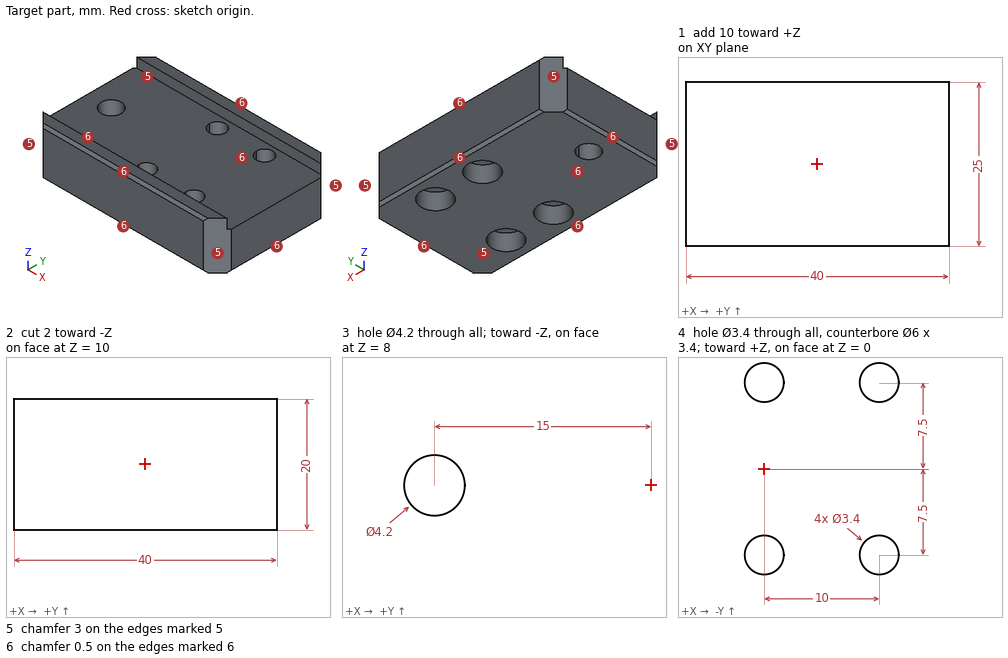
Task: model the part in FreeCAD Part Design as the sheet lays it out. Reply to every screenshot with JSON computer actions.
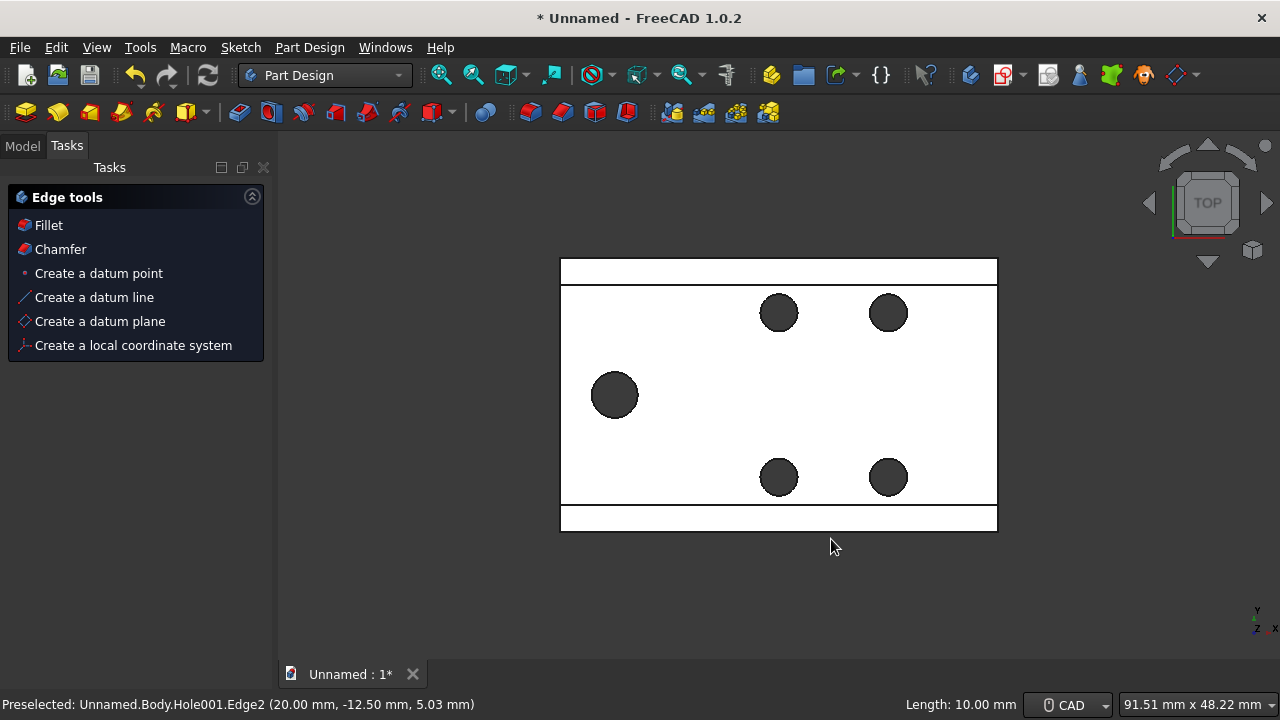
{"action": "key", "text": "1"}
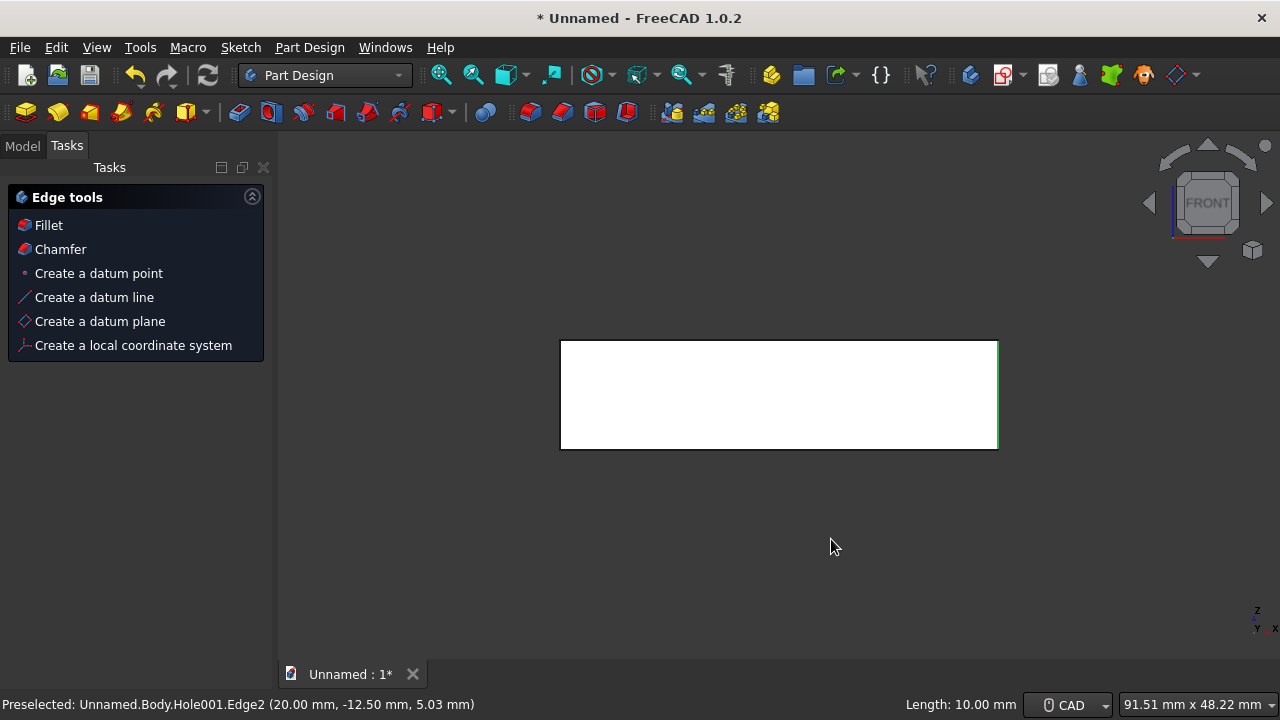
{"action": "left_click", "coordinate": [442, 76]}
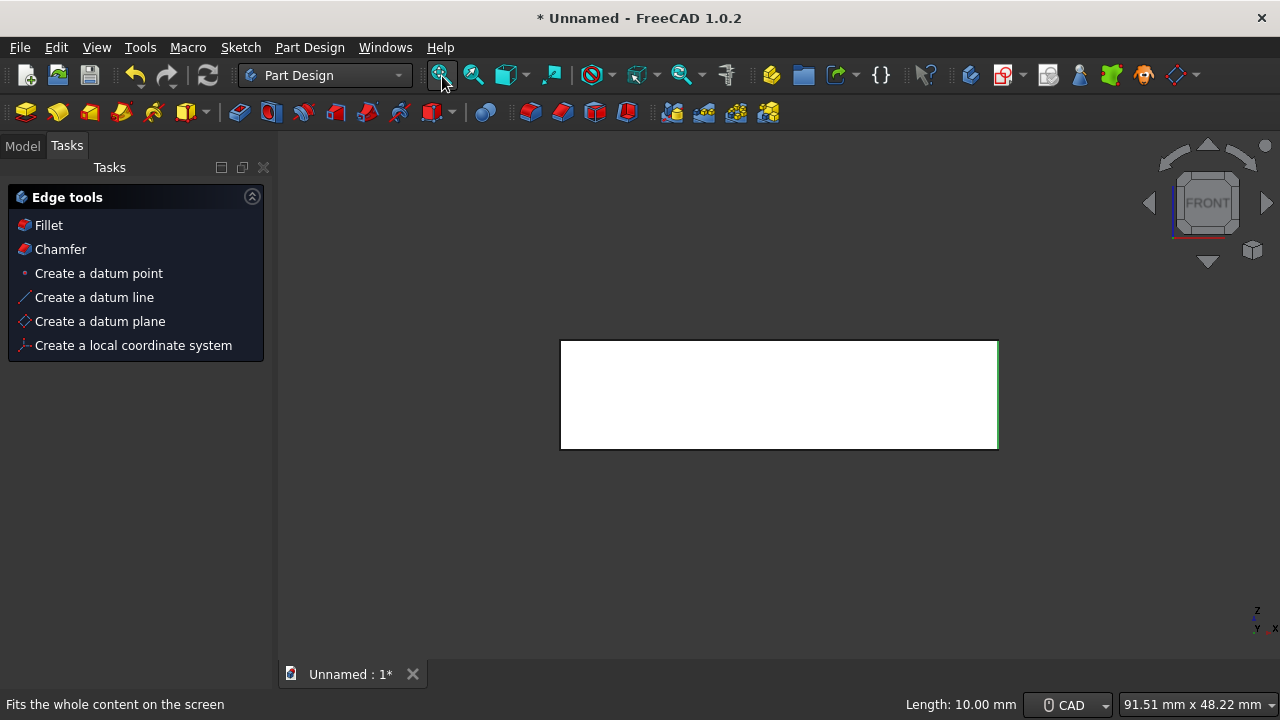
{"action": "left_click", "coordinate": [560, 394], "text": "ctrl"}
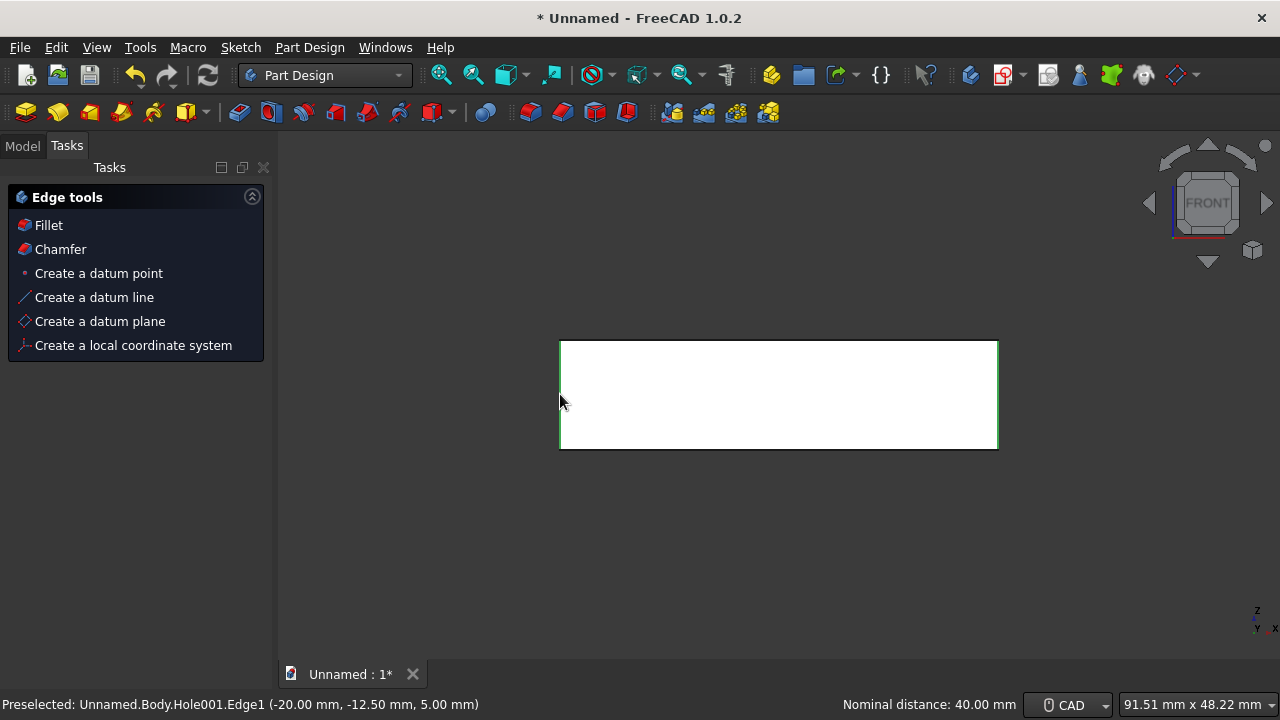
{"action": "key", "text": "3"}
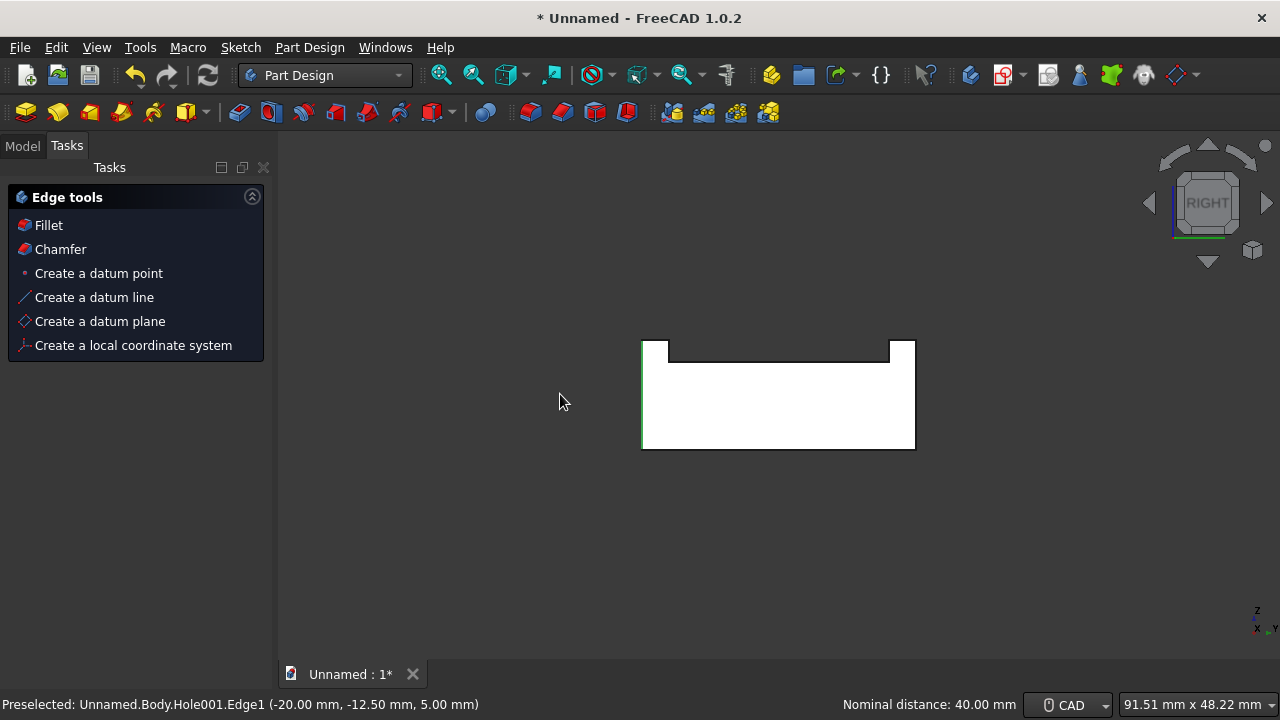
{"action": "left_click", "coordinate": [442, 76]}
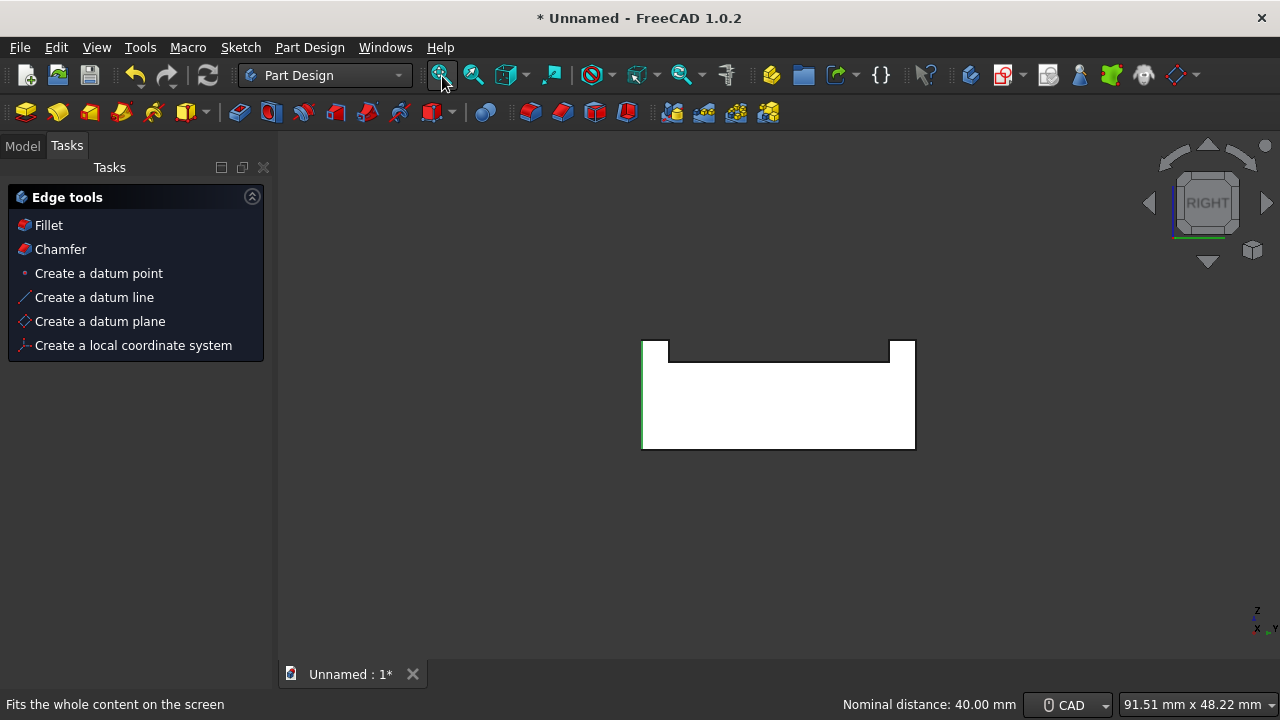
{"action": "left_click", "coordinate": [916, 394], "text": "ctrl"}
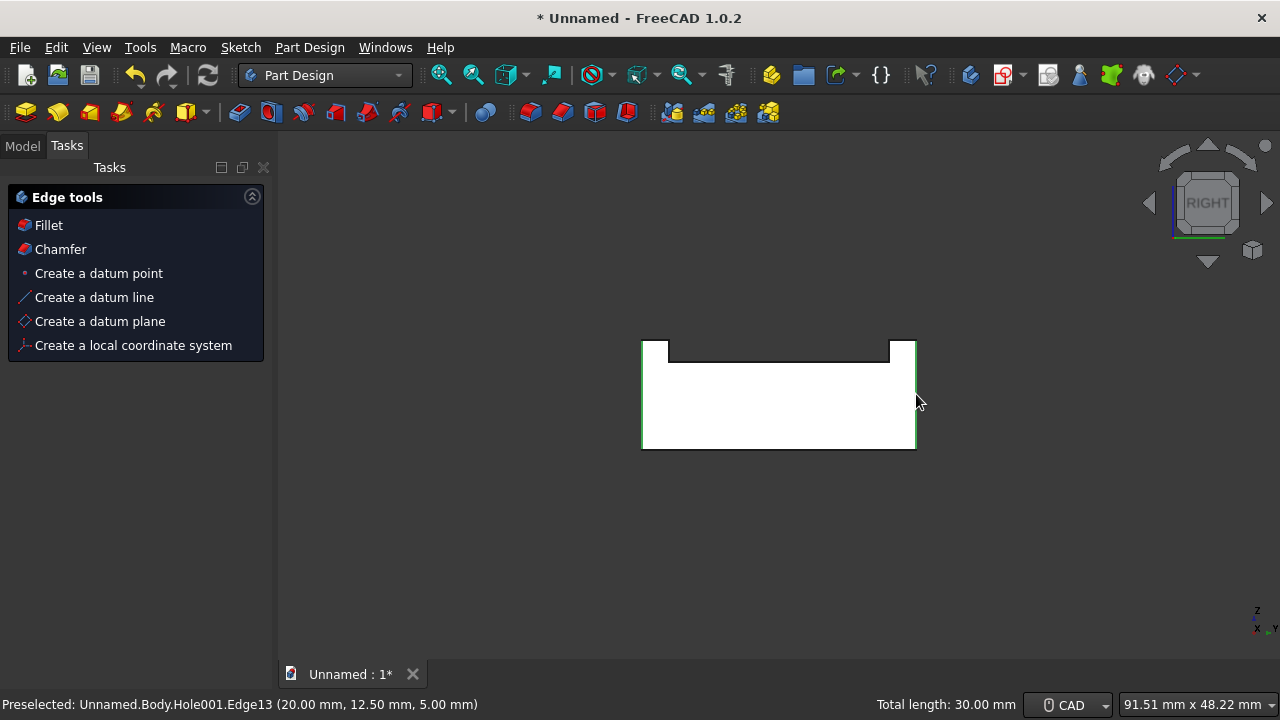
{"action": "key", "text": "5"}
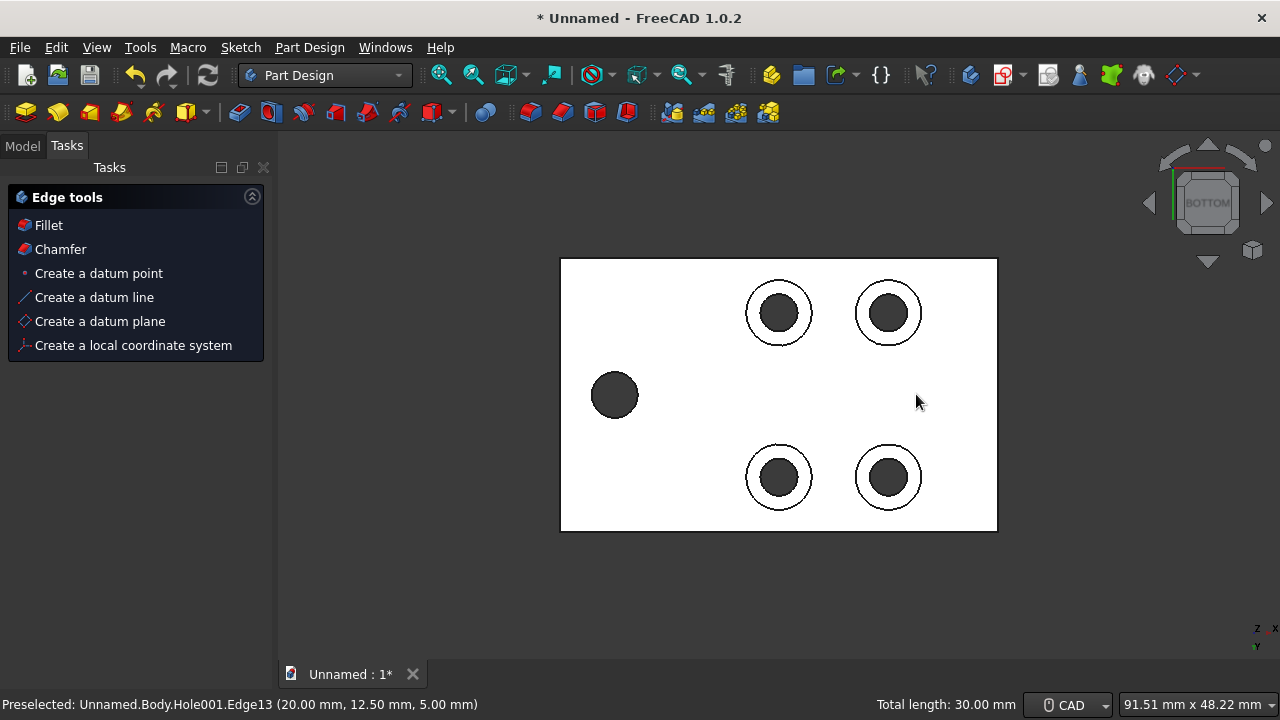
{"action": "key", "text": "4"}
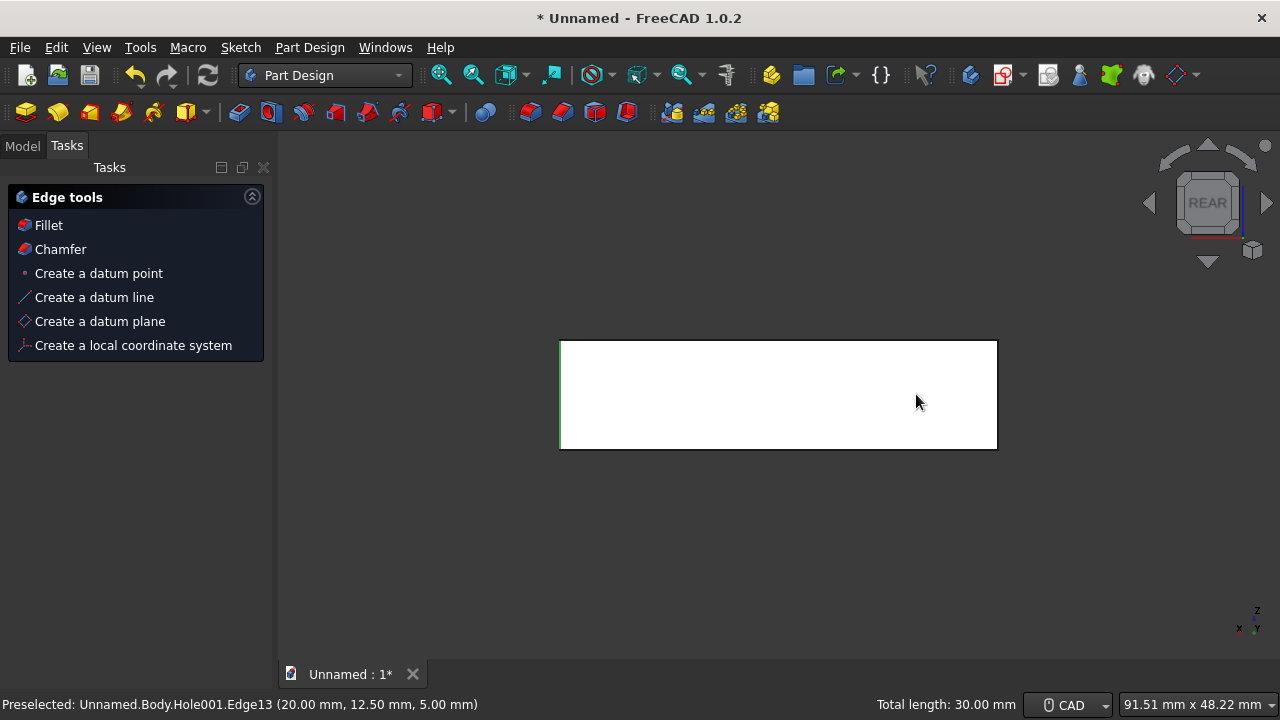
{"action": "left_click", "coordinate": [442, 76]}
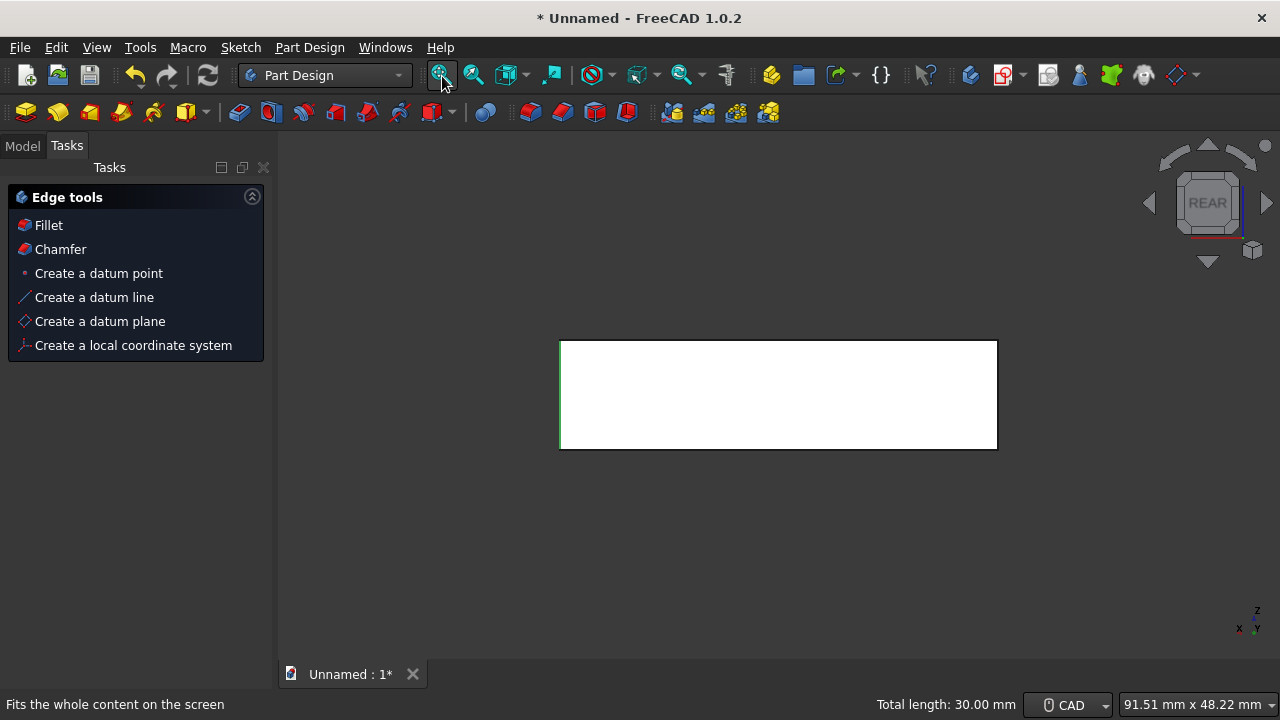
{"action": "left_click", "coordinate": [998, 394], "text": "ctrl"}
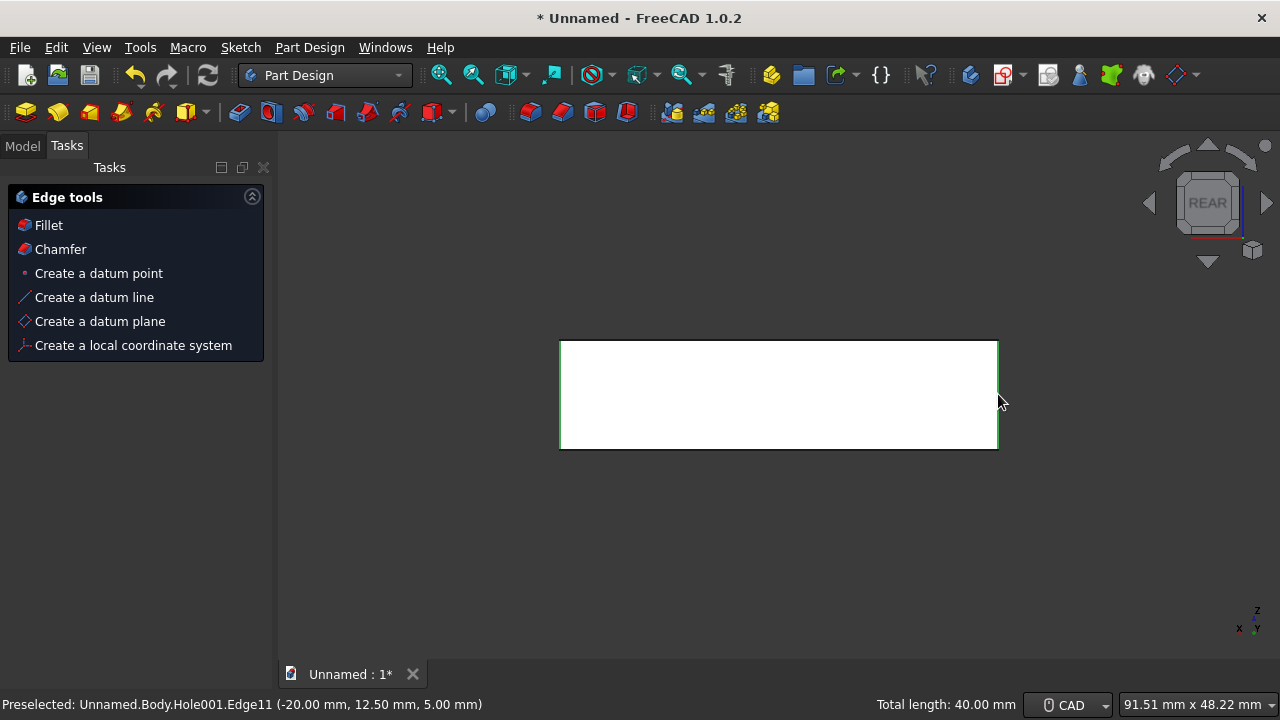
{"action": "left_click", "coordinate": [564, 112]}